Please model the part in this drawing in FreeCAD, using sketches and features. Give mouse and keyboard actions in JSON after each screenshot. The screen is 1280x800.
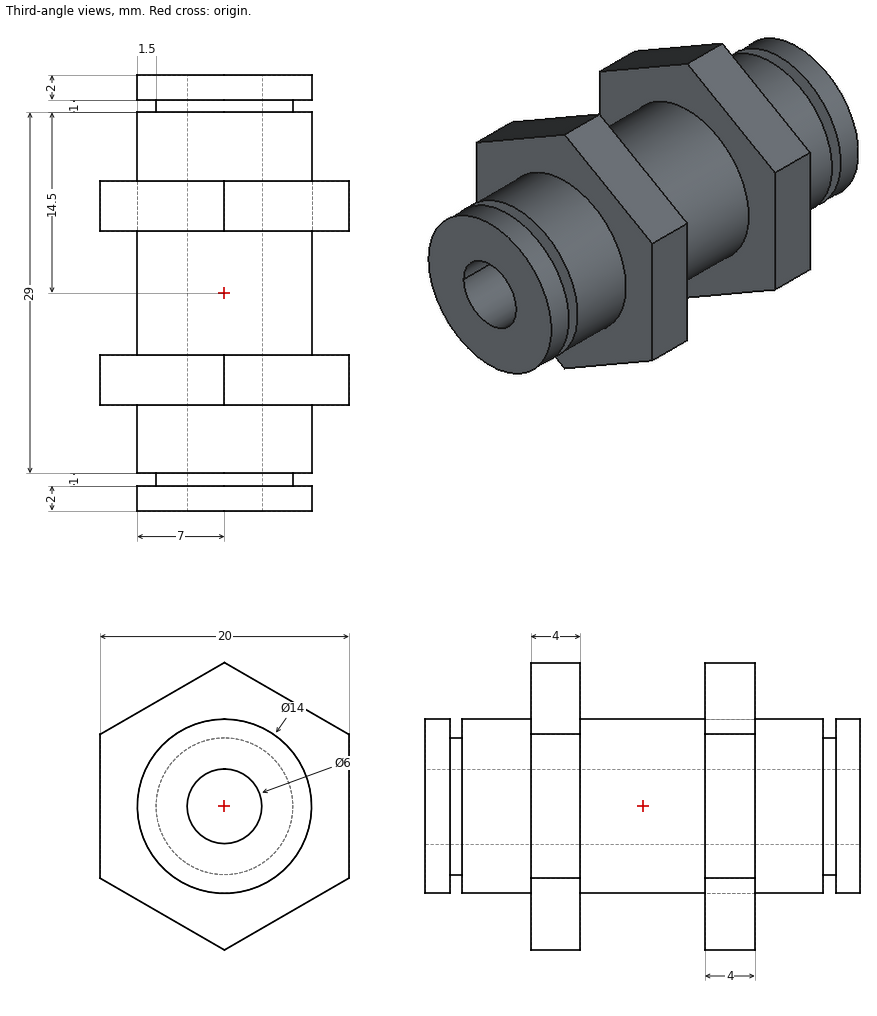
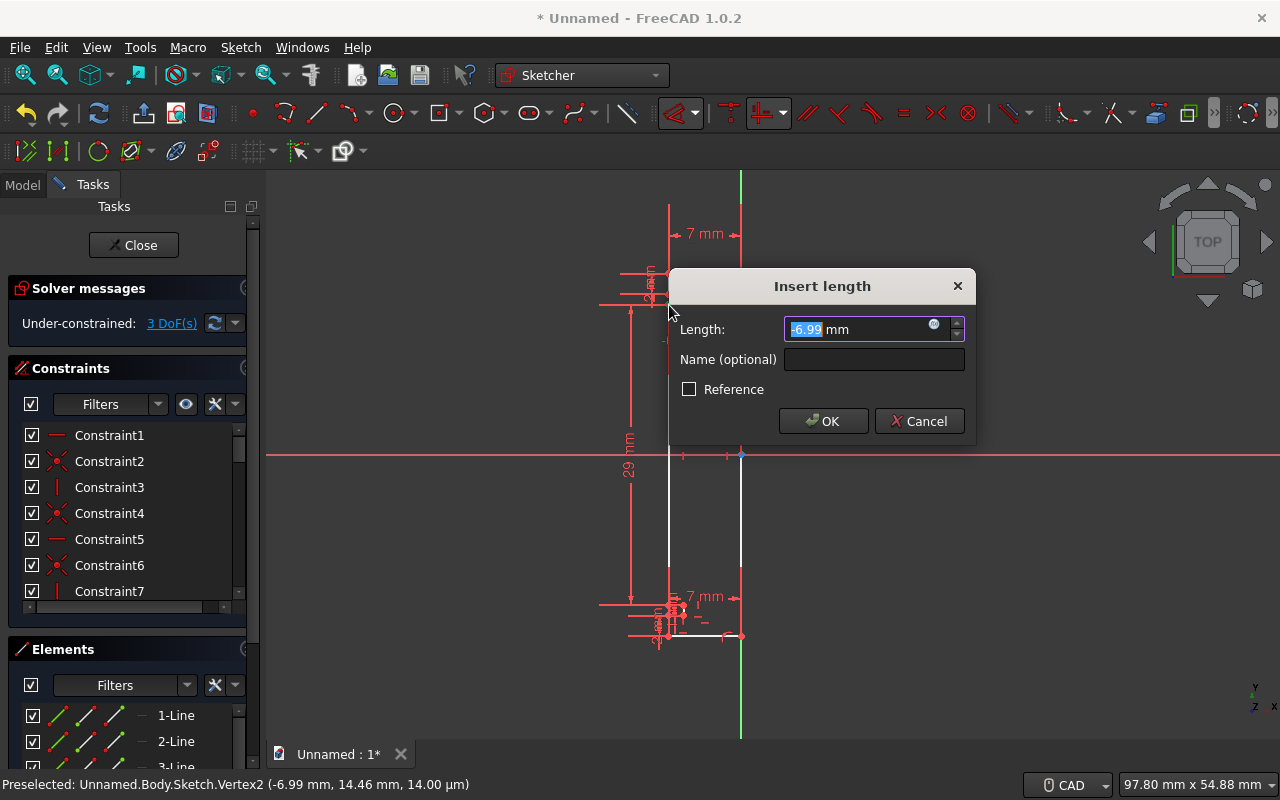
{"action": "type", "text": "-7"}
{"action": "key", "text": "Return"}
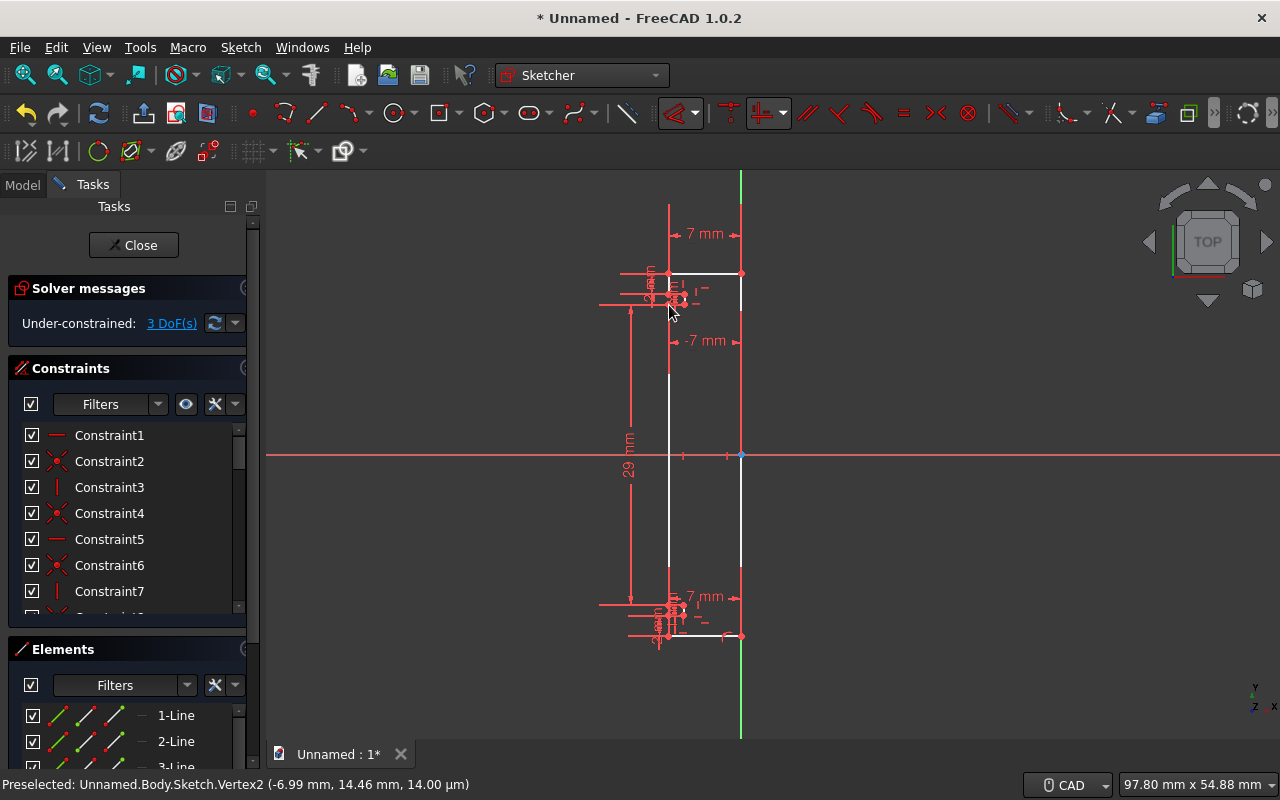
{"action": "scroll", "coordinate": [677, 305], "scroll_direction": "up", "scroll_amount": 5}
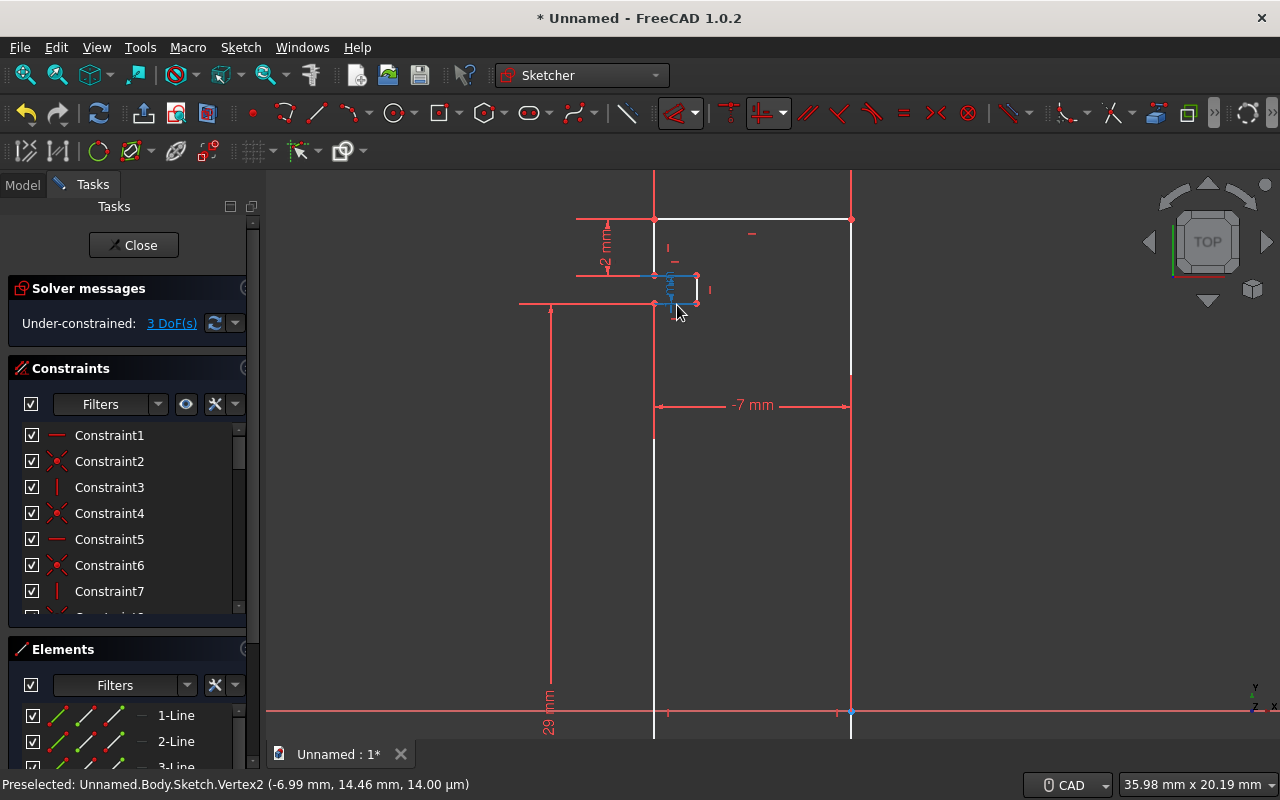
{"action": "left_click", "coordinate": [680, 304]}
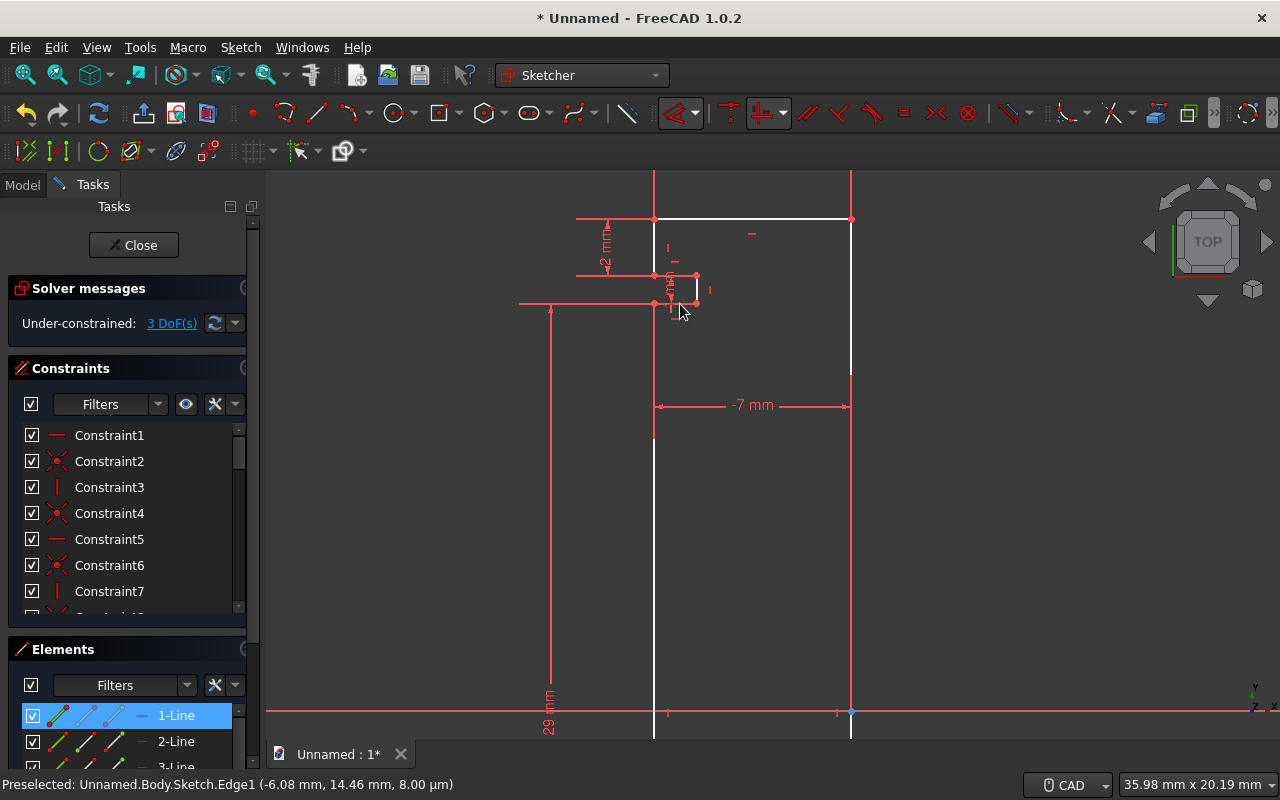
{"action": "key", "text": "l"}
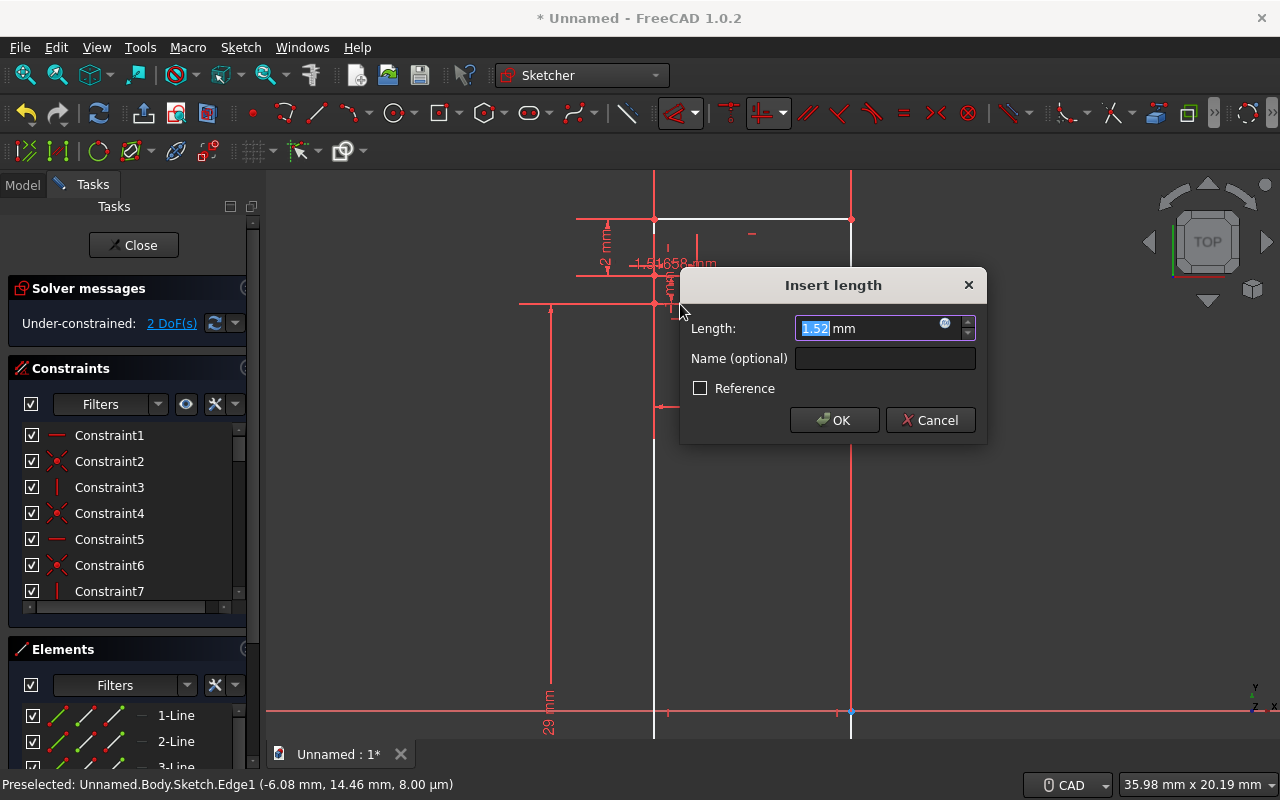
{"action": "type", "text": "1.5"}
{"action": "key", "text": "Return"}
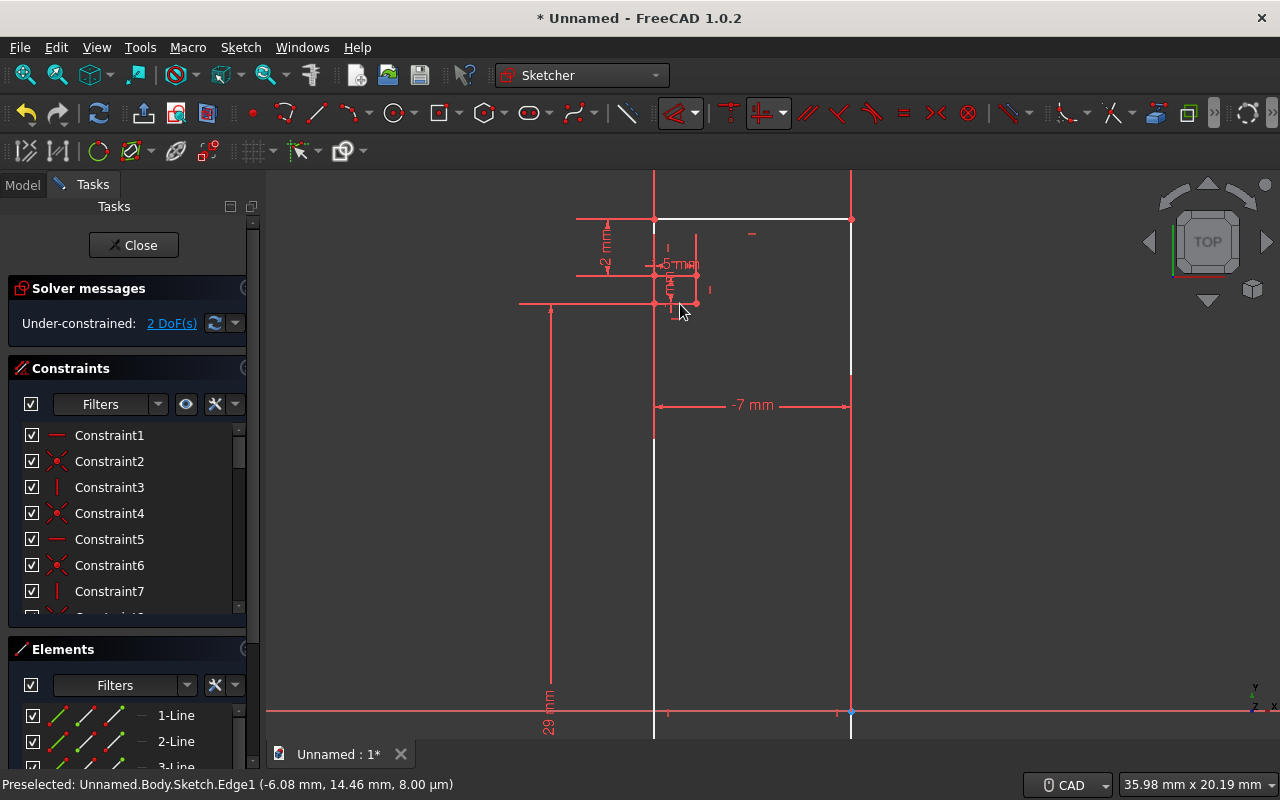
{"action": "scroll", "coordinate": [676, 305], "scroll_direction": "down", "scroll_amount": 5}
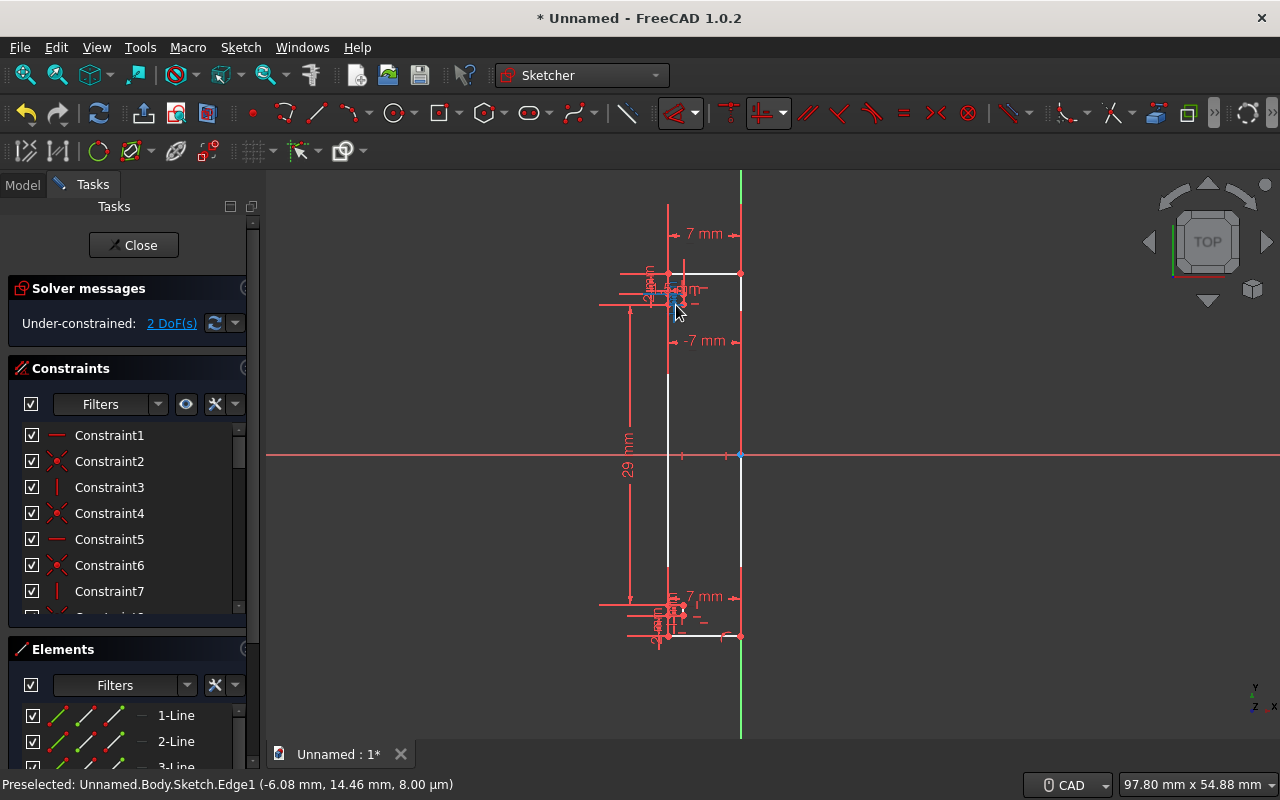
{"action": "scroll", "coordinate": [673, 605], "scroll_direction": "up", "scroll_amount": 6}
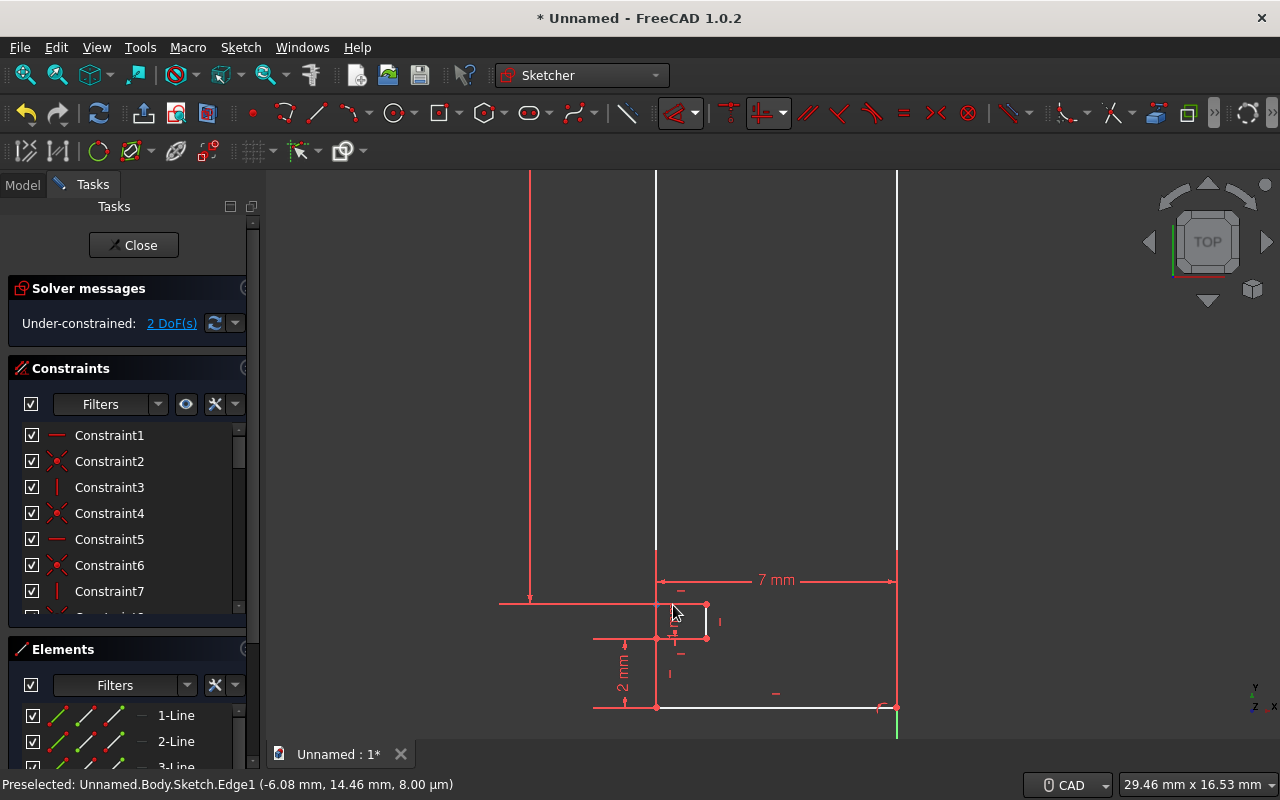
{"action": "left_click", "coordinate": [691, 604]}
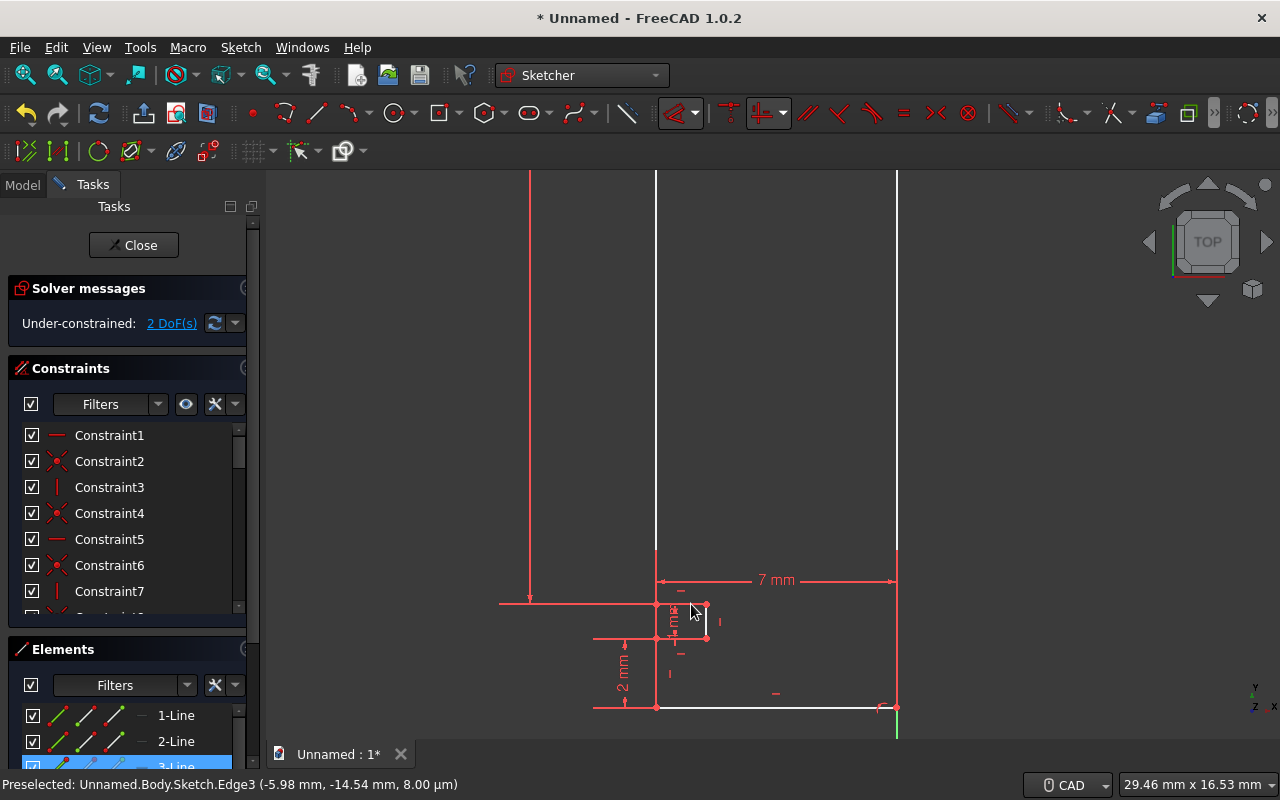
{"action": "left_click", "coordinate": [698, 114]}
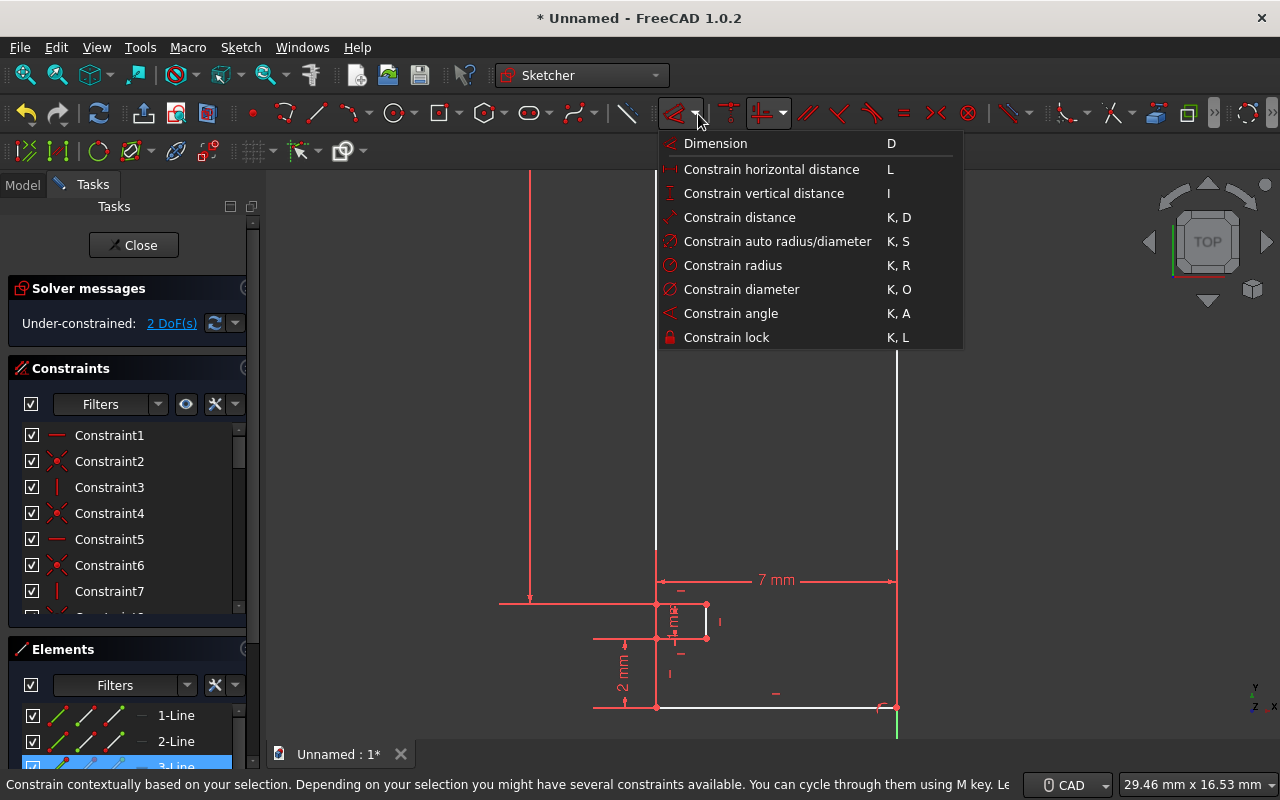
{"action": "left_click", "coordinate": [811, 169]}